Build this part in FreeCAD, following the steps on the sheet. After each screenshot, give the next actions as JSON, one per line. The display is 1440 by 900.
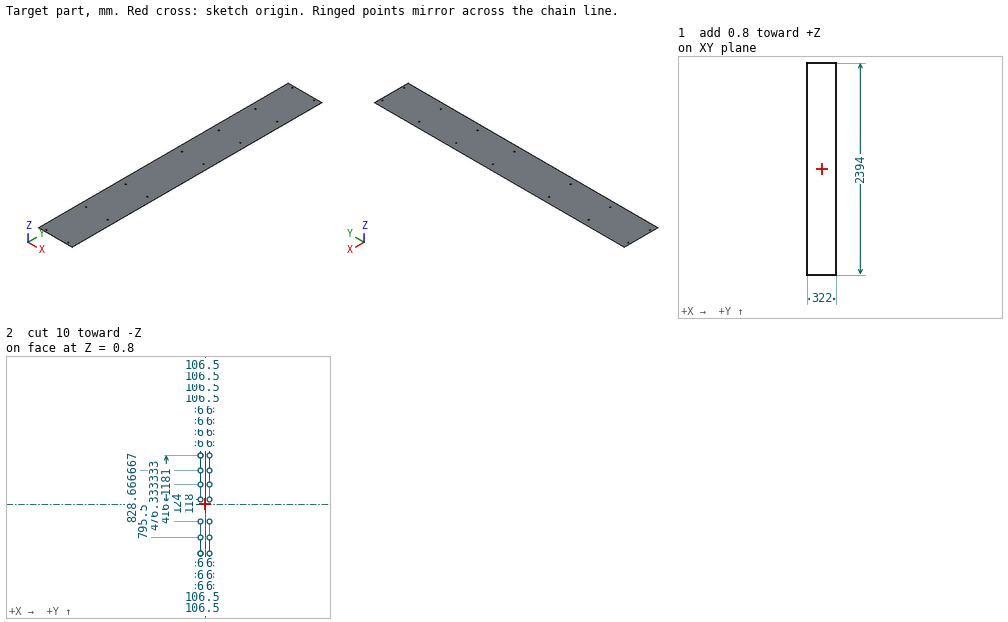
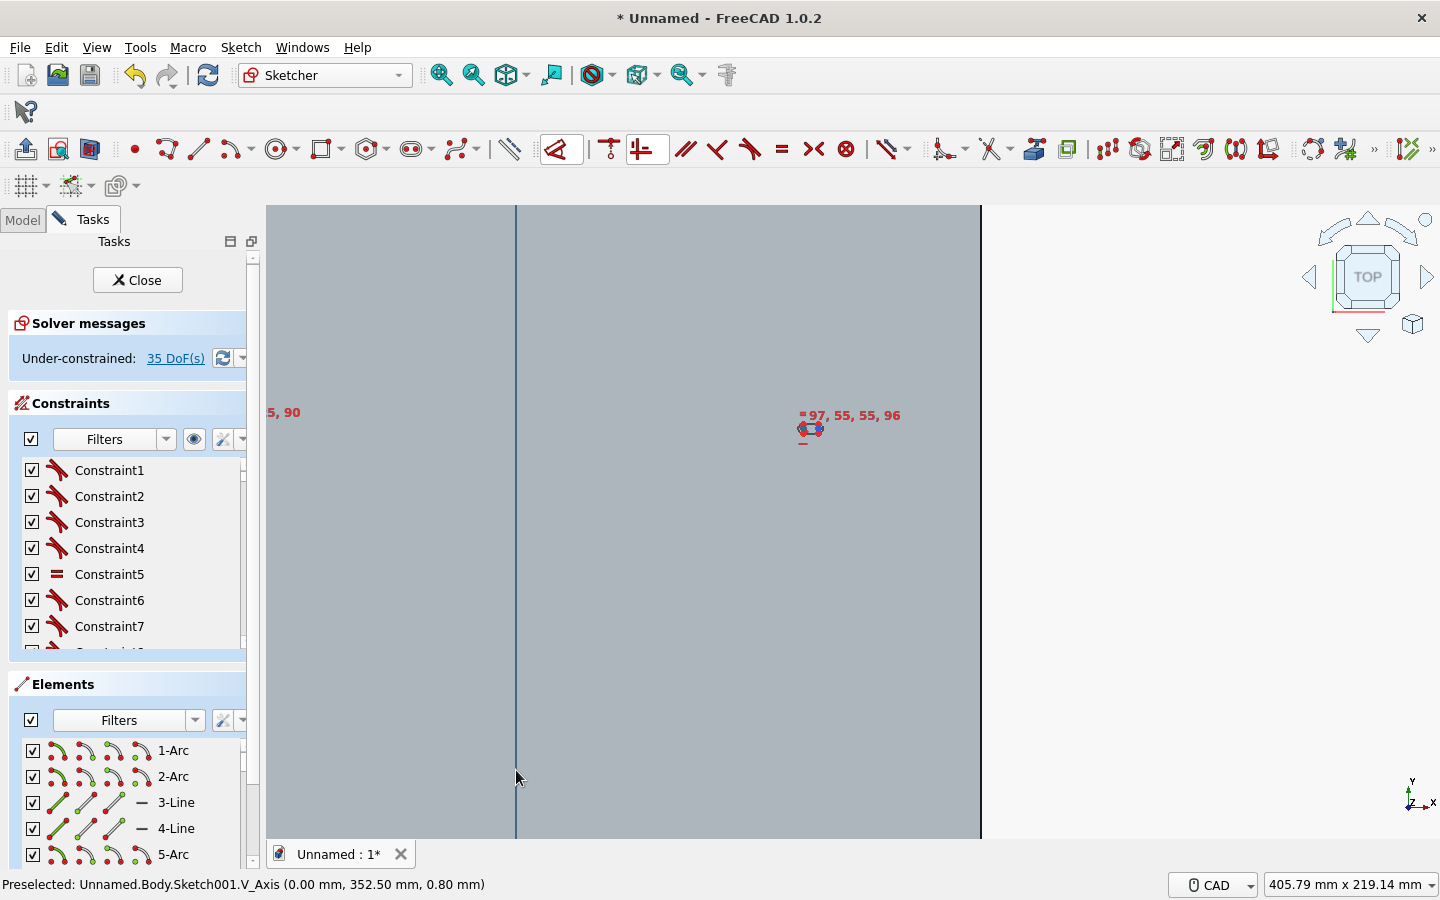
{"action": "key", "text": "s"}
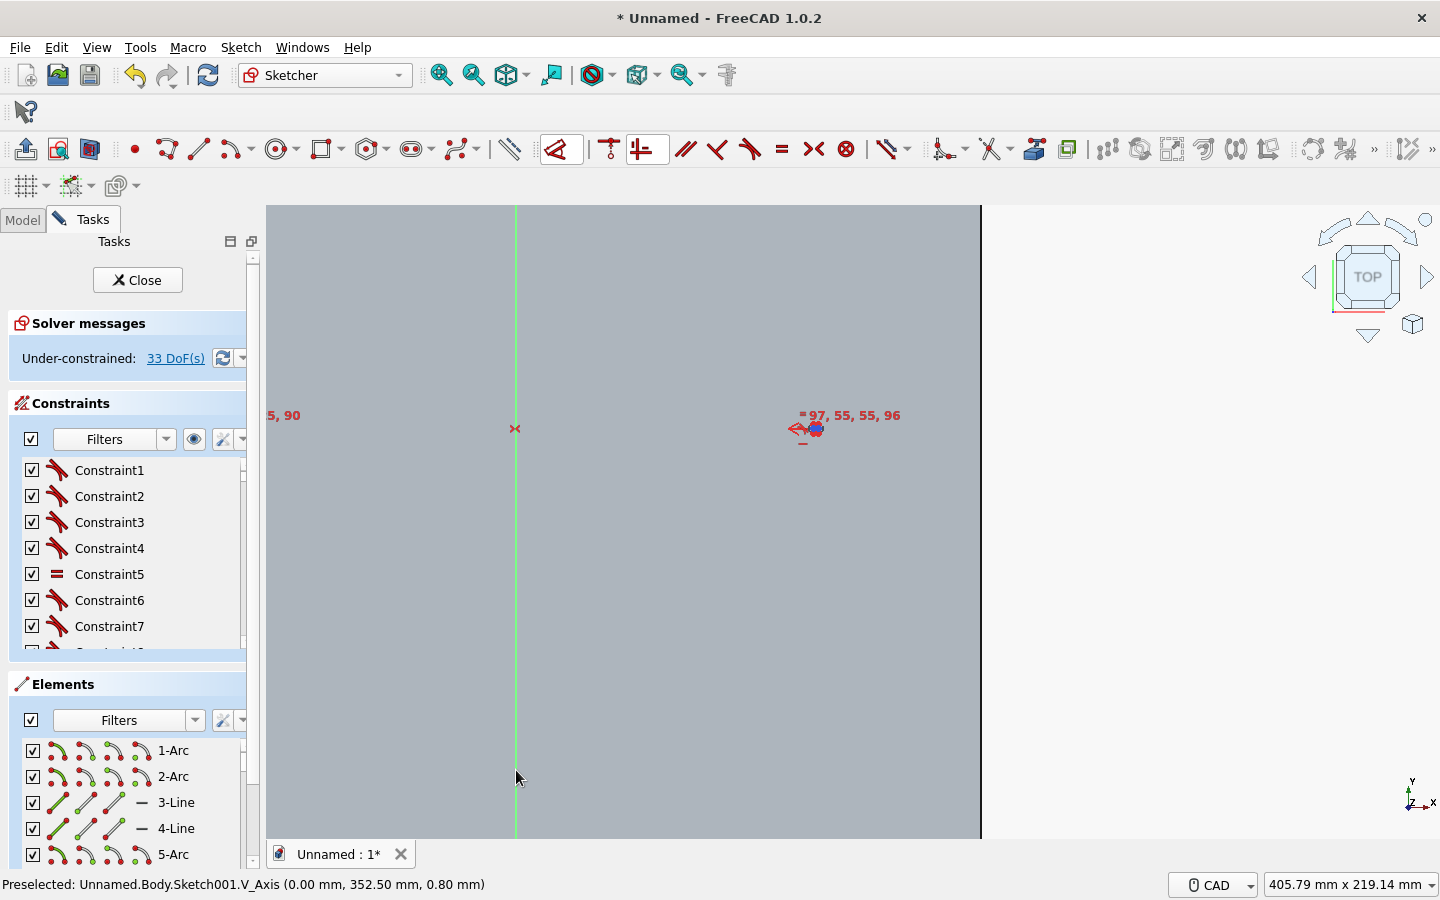
{"action": "scroll", "coordinate": [802, 440], "scroll_direction": "down", "scroll_amount": 14}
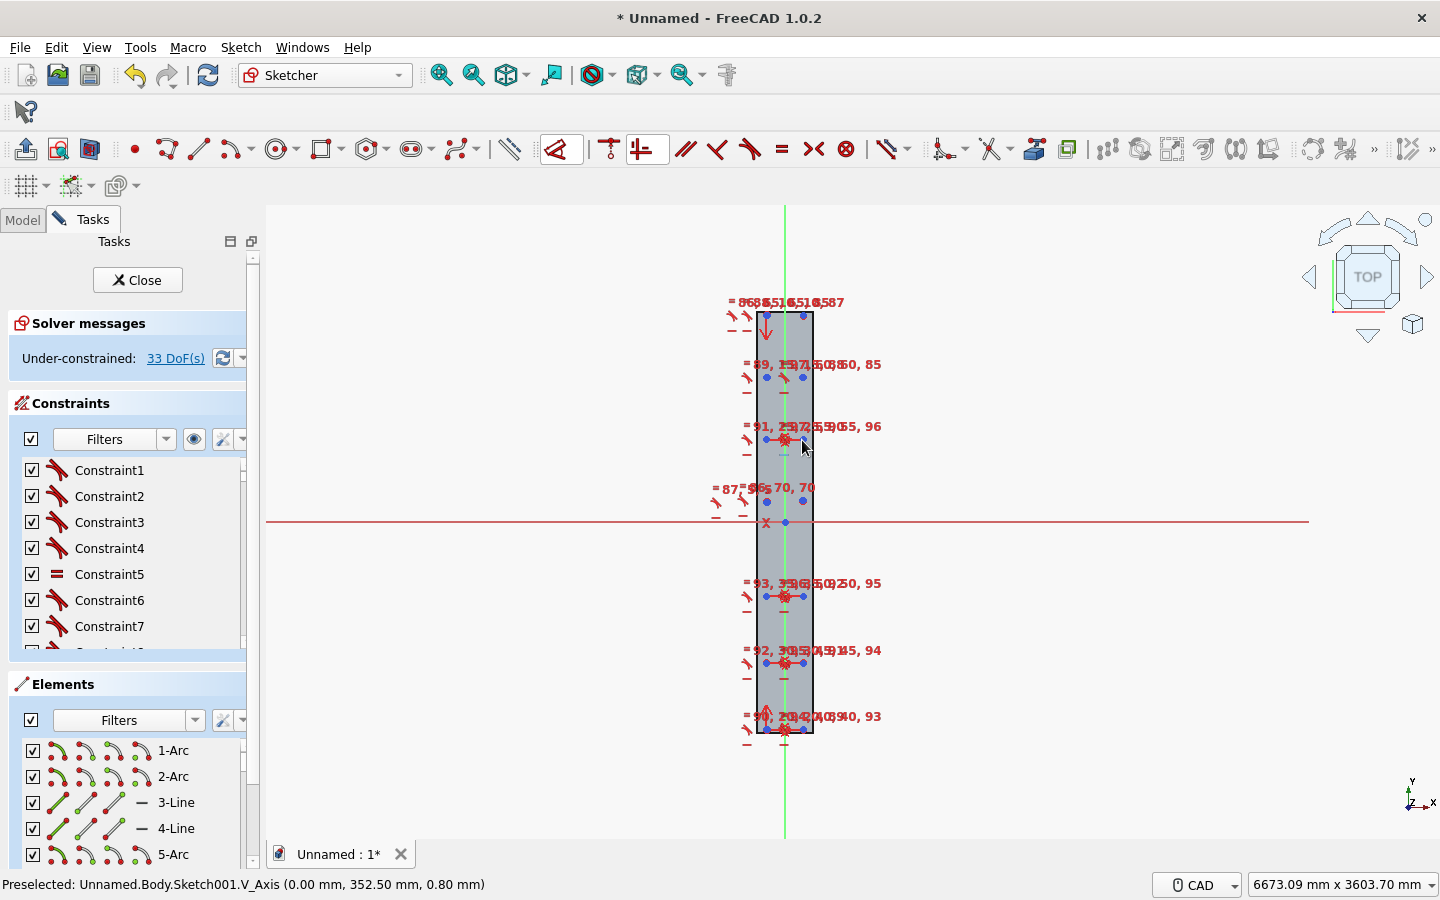
{"action": "scroll", "coordinate": [767, 378], "scroll_direction": "up", "scroll_amount": 14}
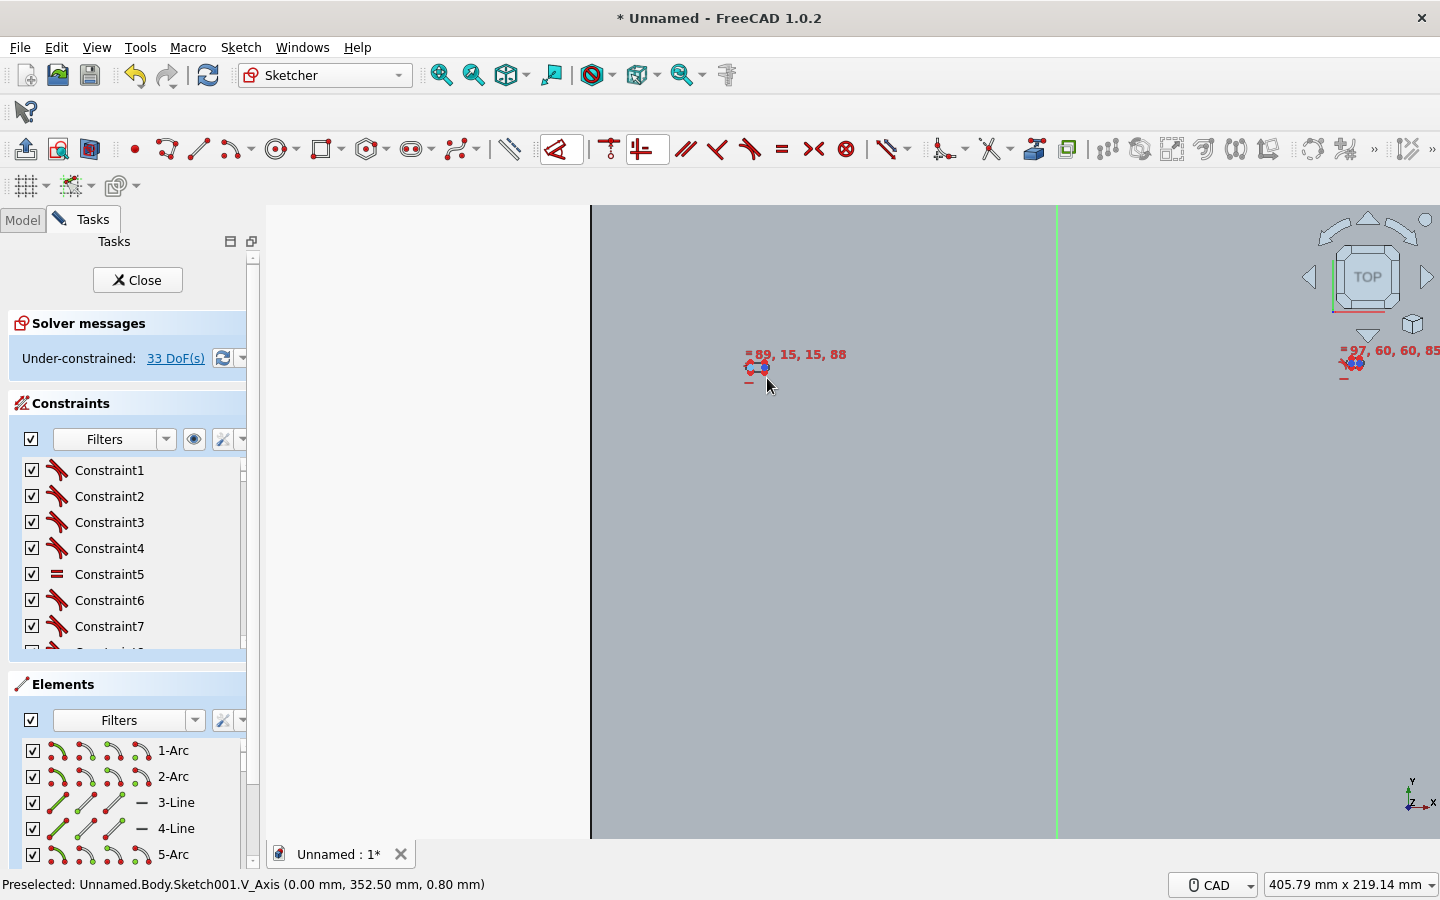
{"action": "left_click", "coordinate": [764, 367]}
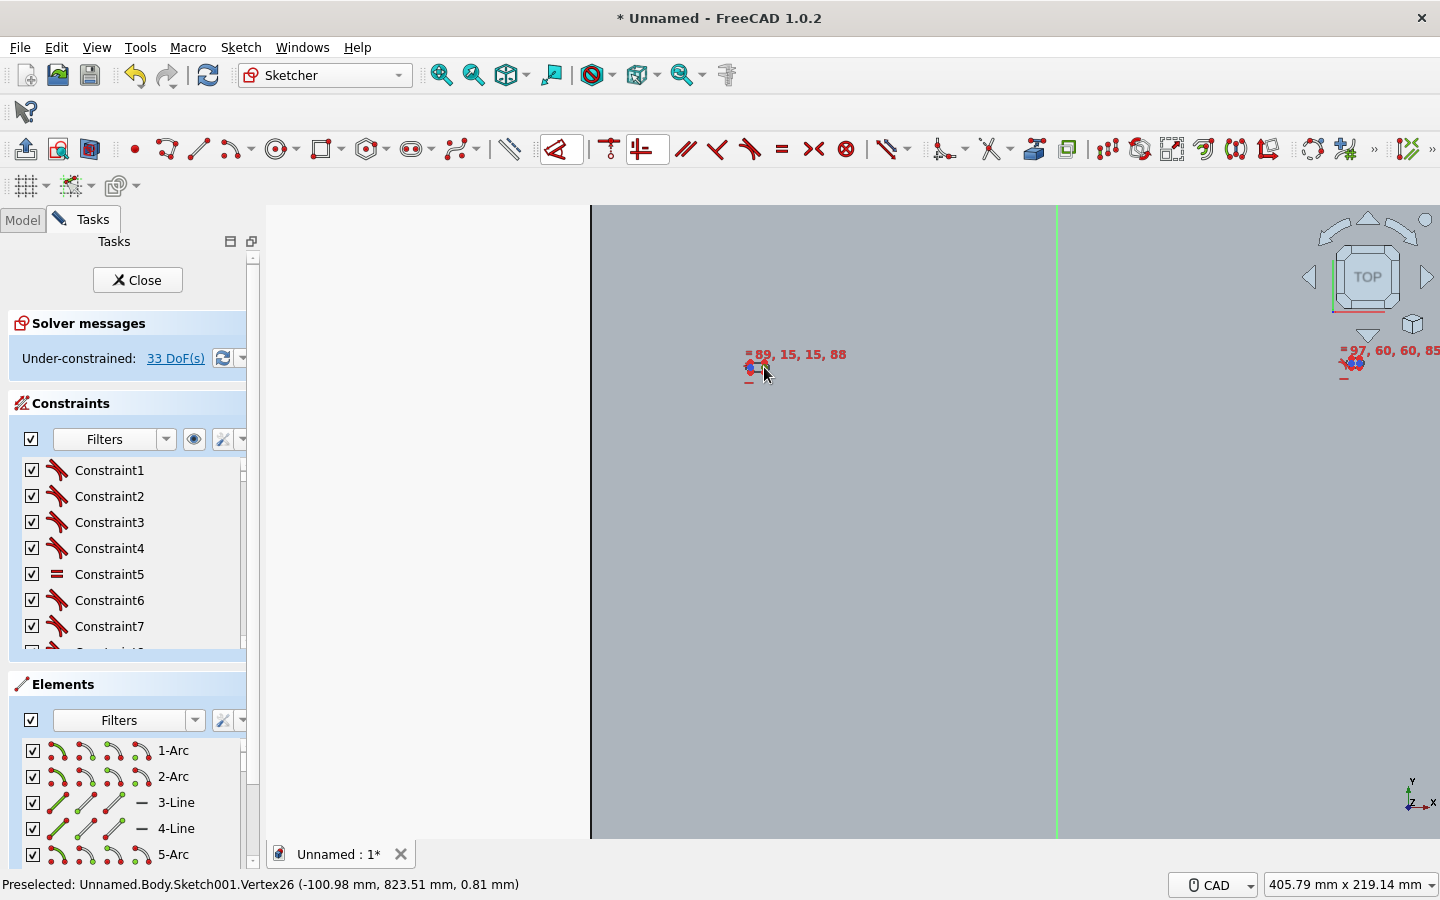
{"action": "scroll", "coordinate": [767, 378], "scroll_direction": "down", "scroll_amount": 14}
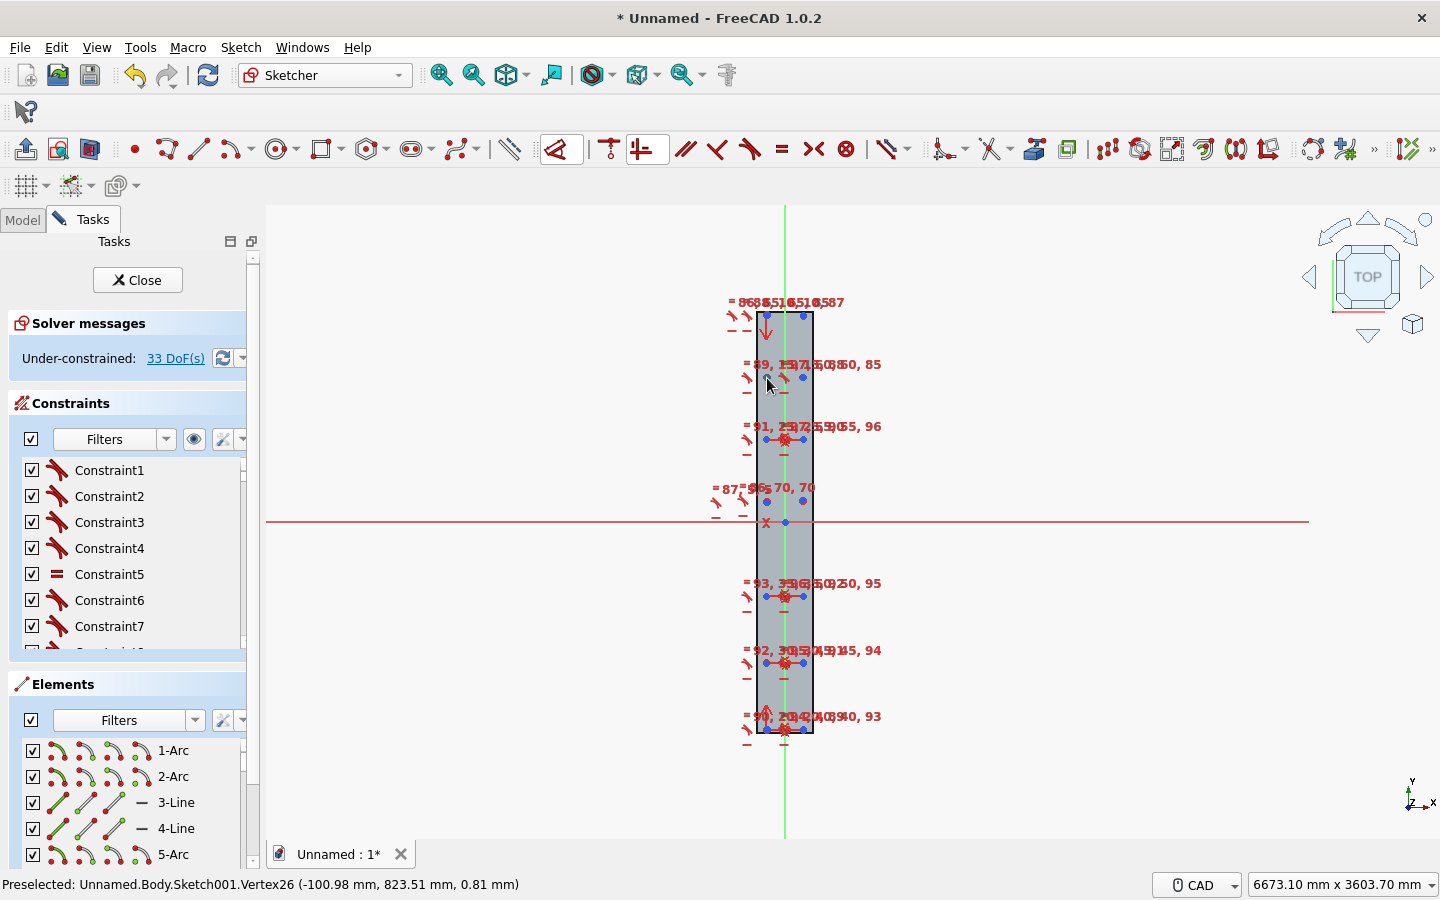
{"action": "scroll", "coordinate": [803, 377], "scroll_direction": "up", "scroll_amount": 14}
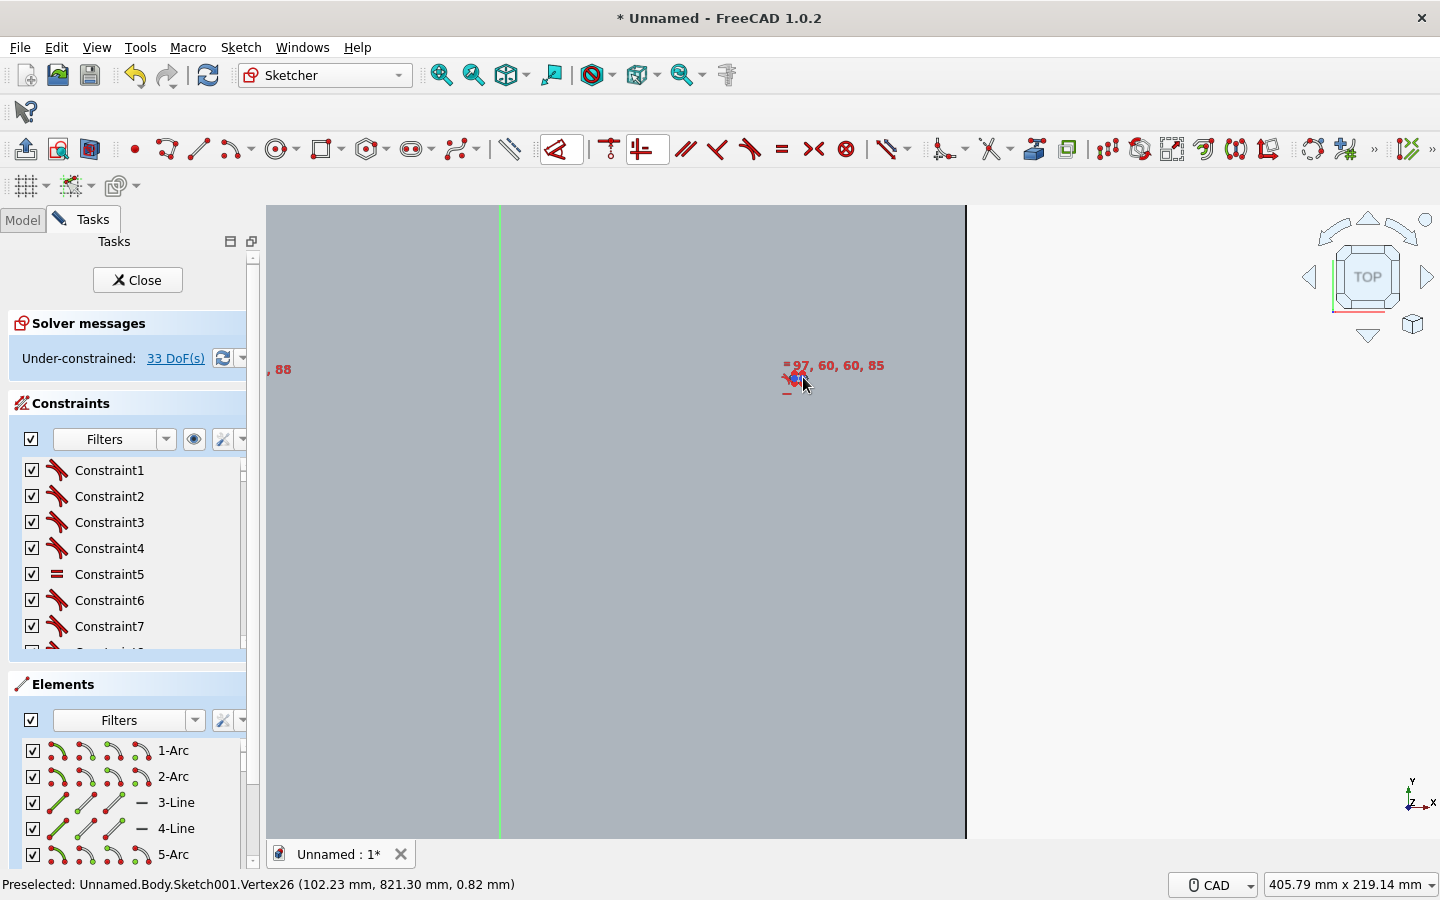
{"action": "scroll", "coordinate": [795, 379], "scroll_direction": "up", "scroll_amount": 4}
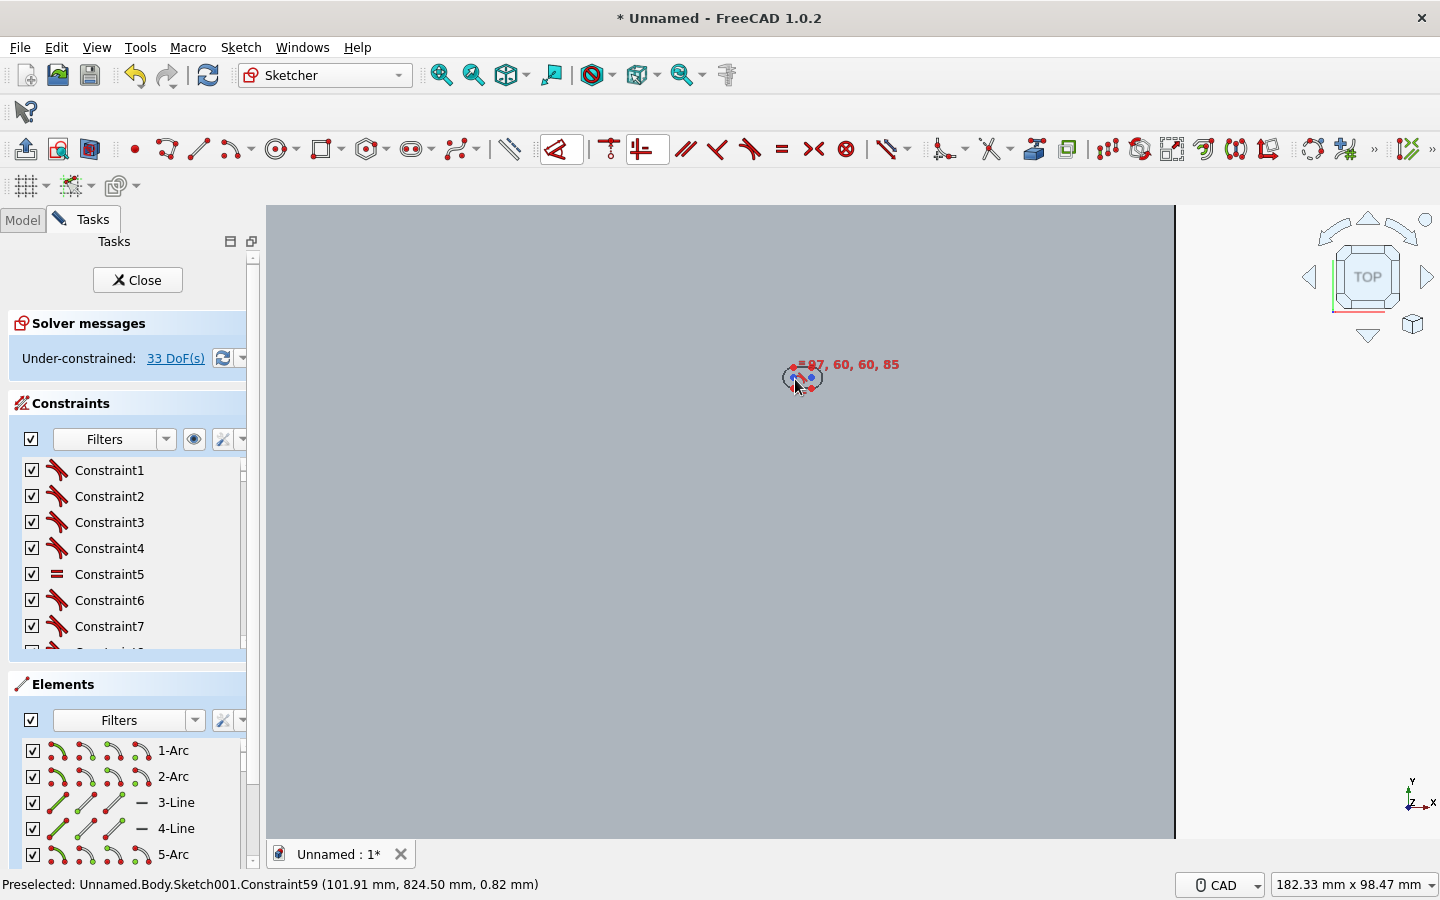
{"action": "left_click", "coordinate": [794, 378]}